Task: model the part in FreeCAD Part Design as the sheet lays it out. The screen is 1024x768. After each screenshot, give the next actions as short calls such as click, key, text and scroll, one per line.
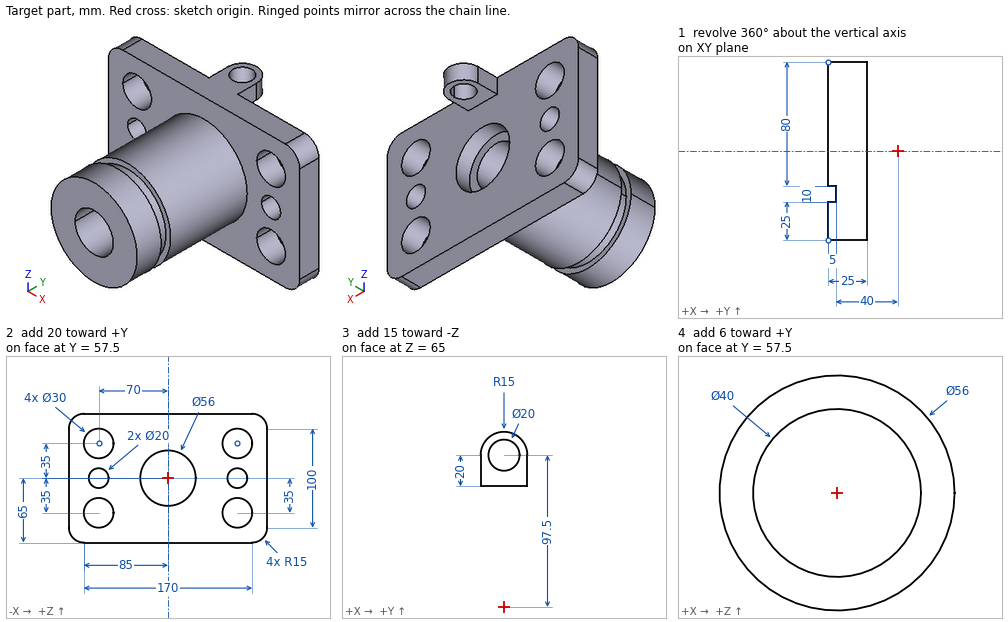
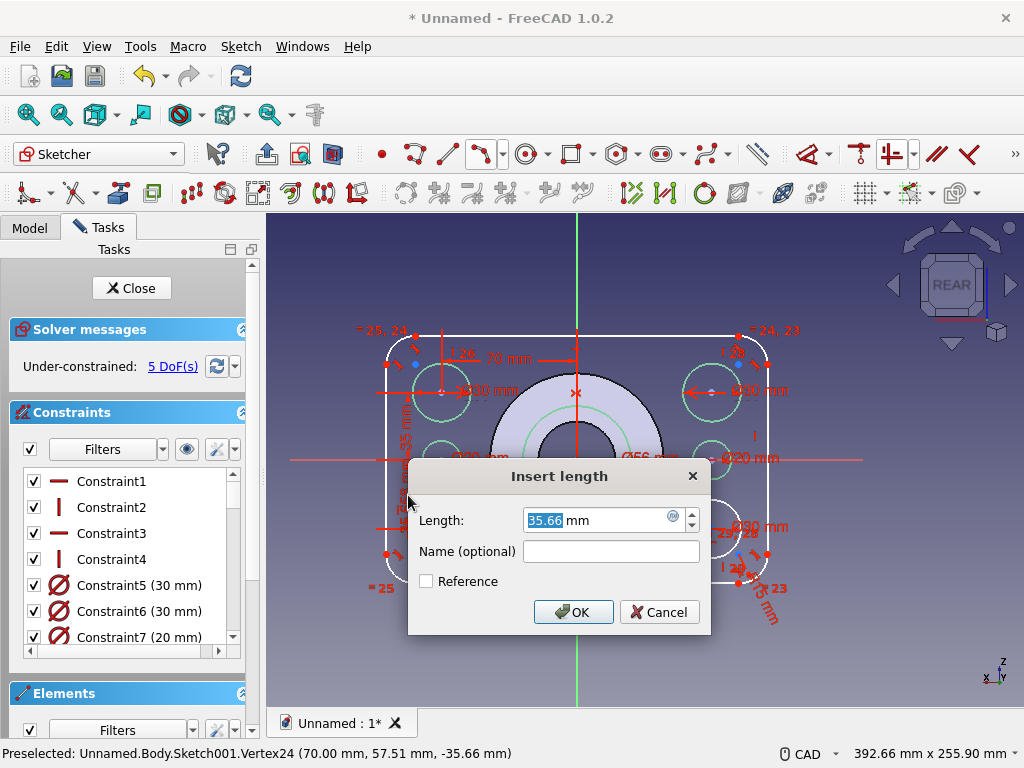
text(35)
key(Return)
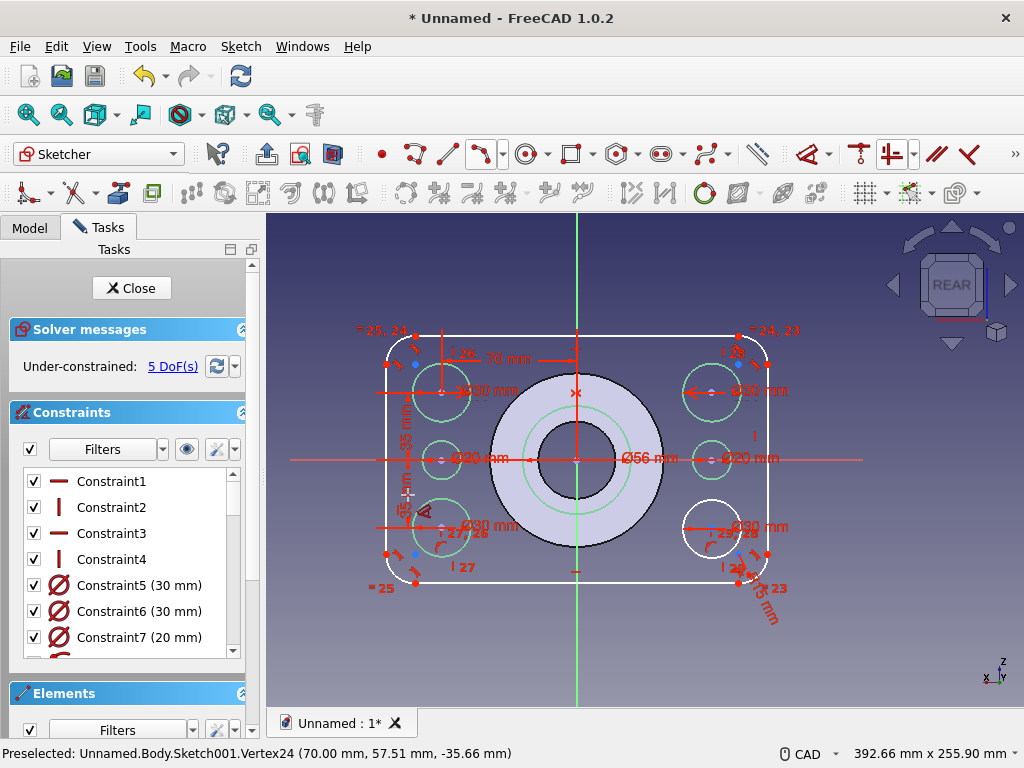
click(712, 529)
click(746, 495)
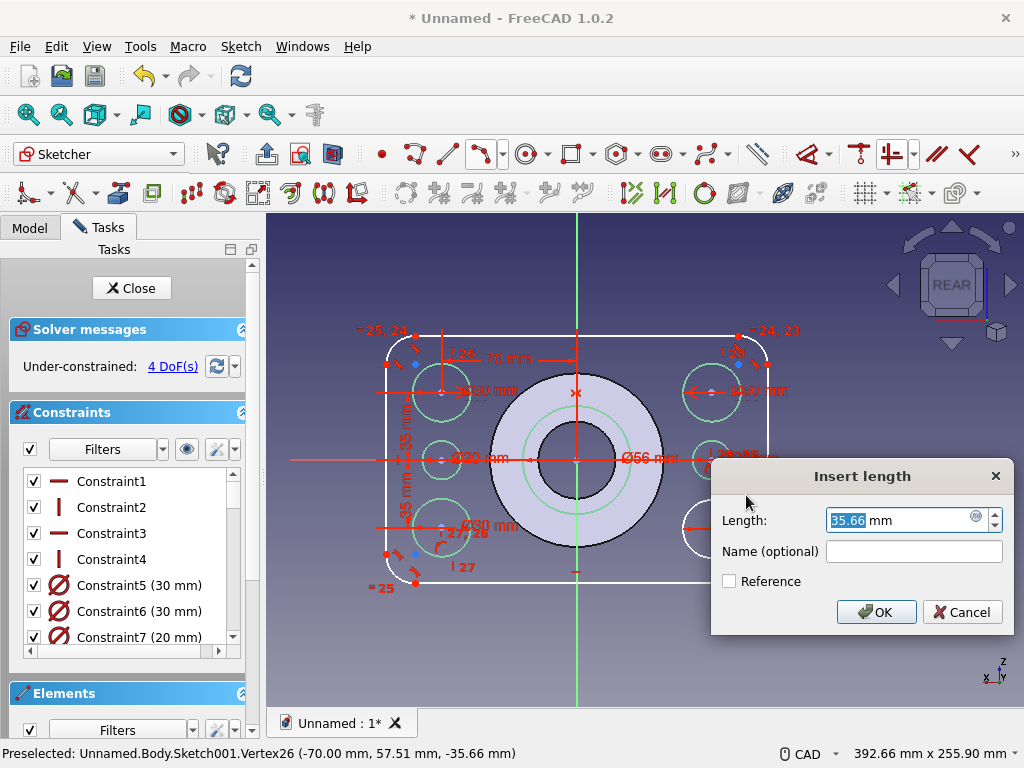
text(35)
key(Return)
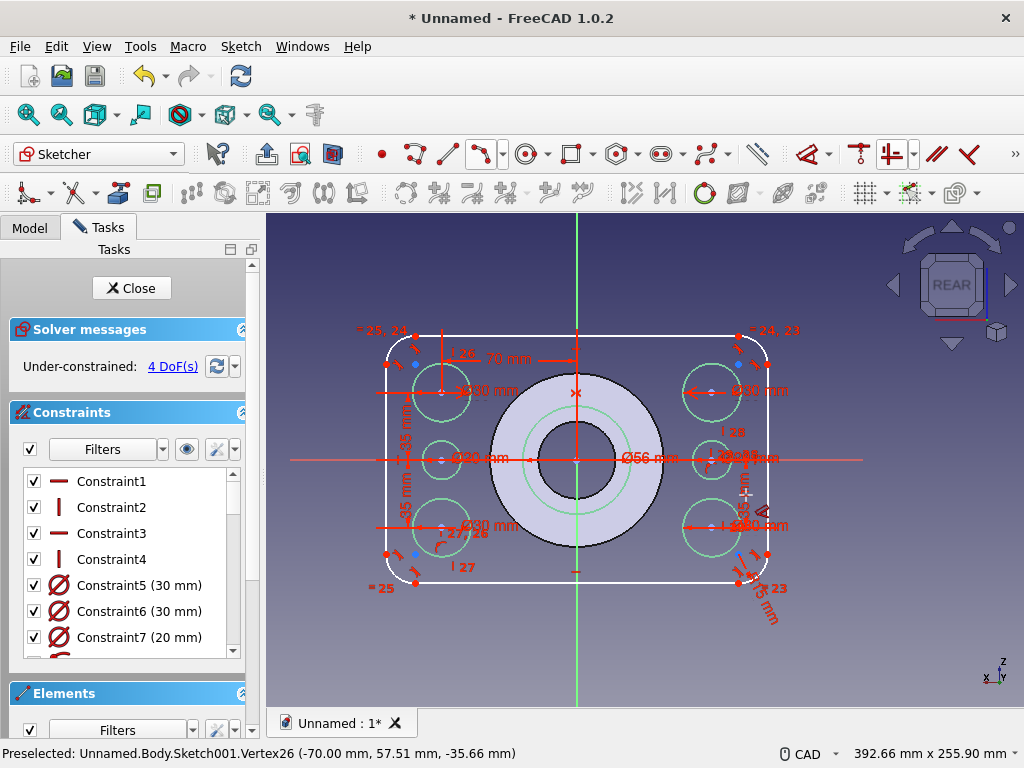
click(512, 583)
click(503, 617)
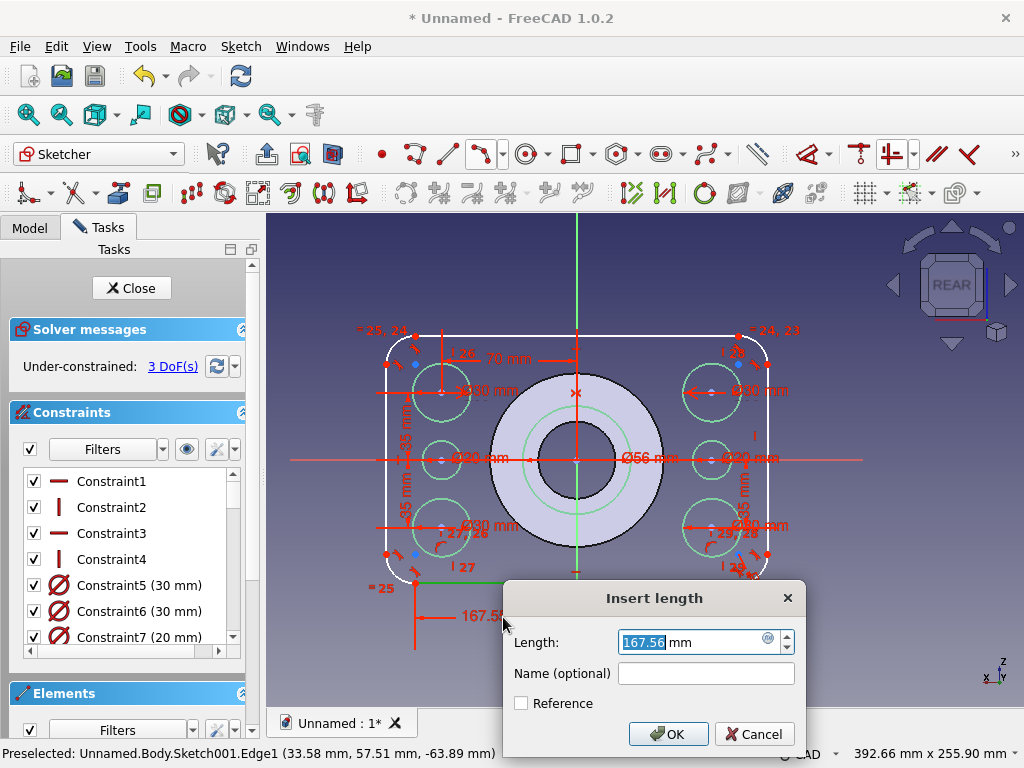
text(170)
key(Return)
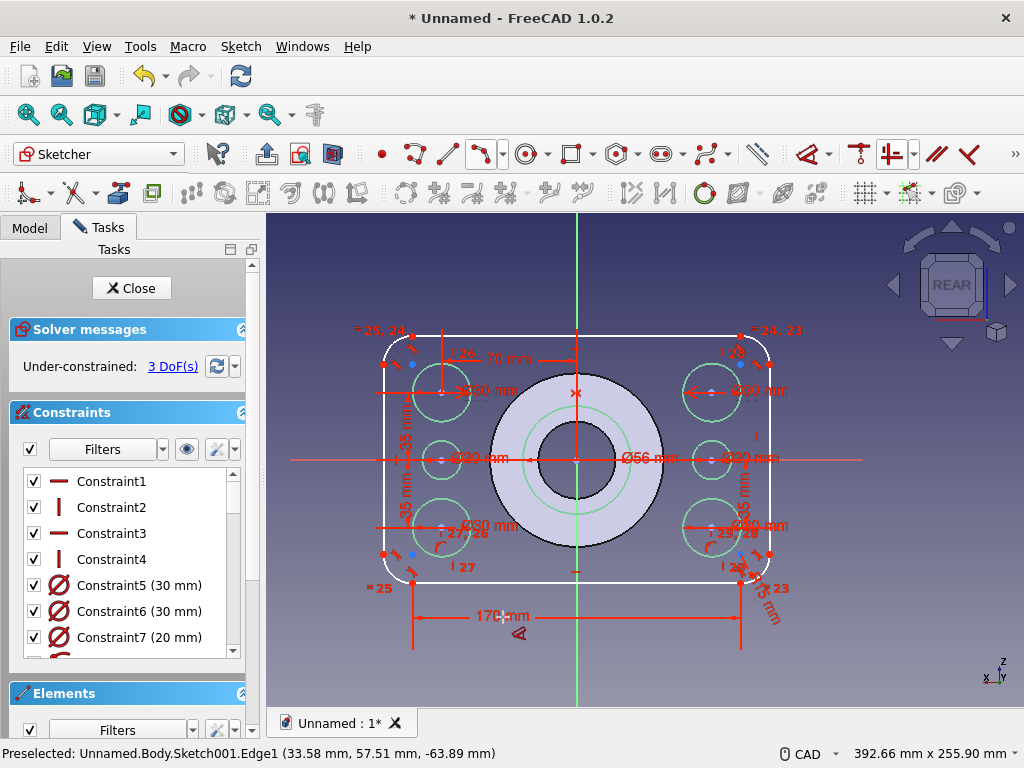
click(770, 498)
click(804, 416)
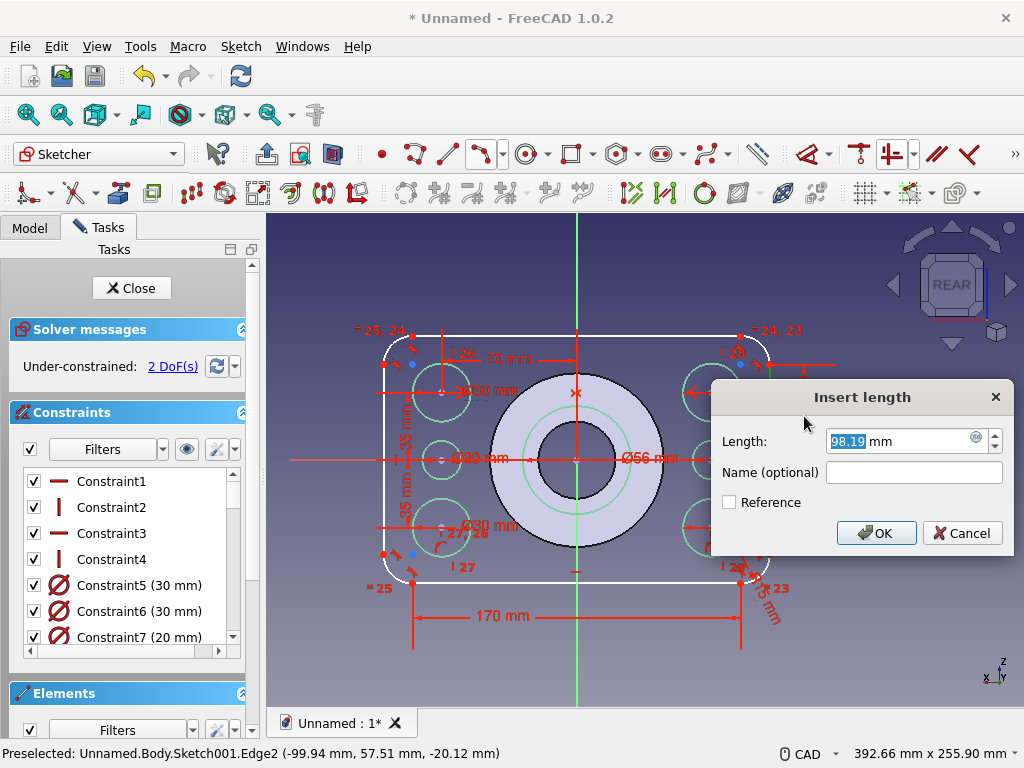
text(100)
key(Return)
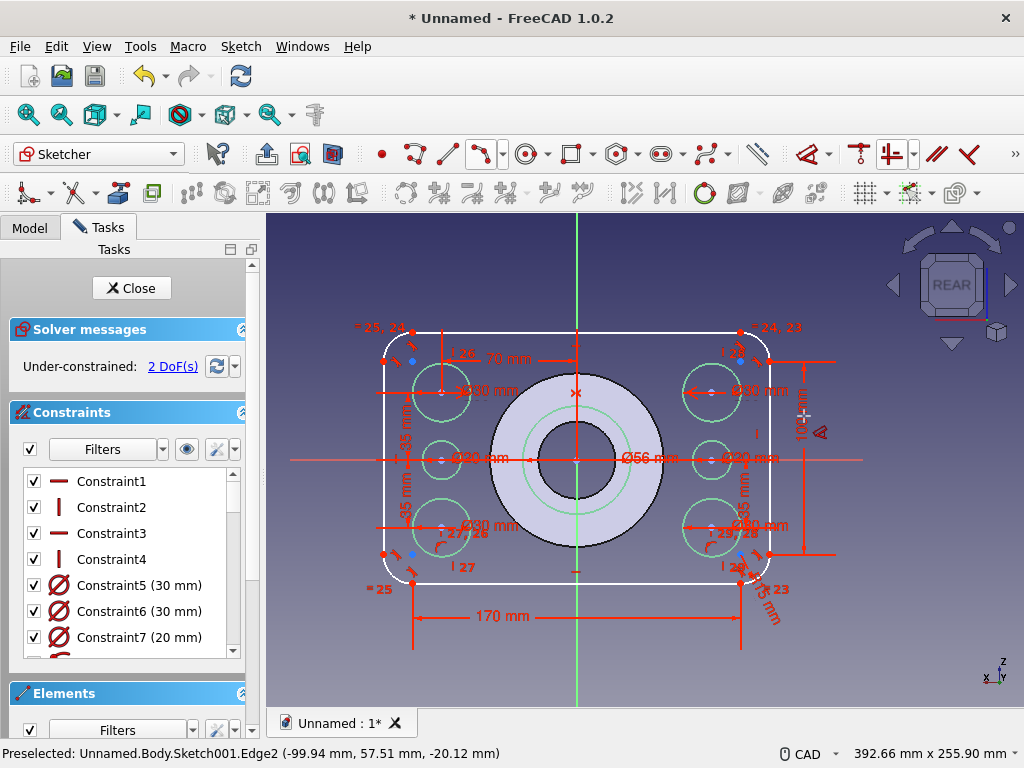
click(413, 584)
click(495, 426)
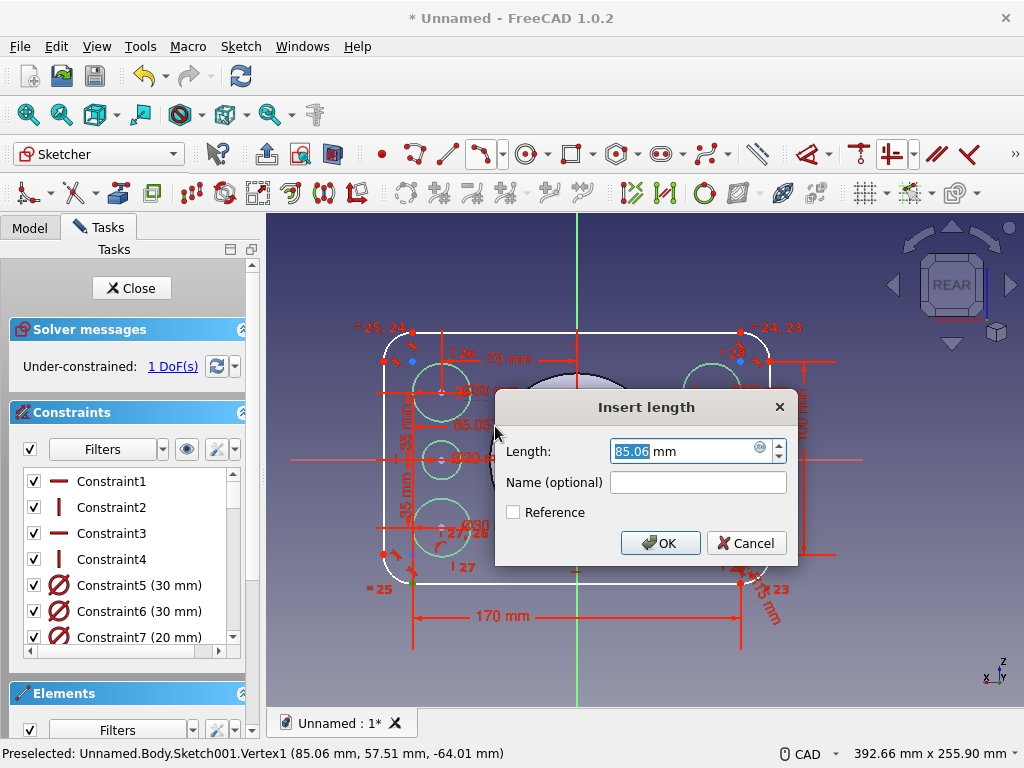
text(85)
key(Return)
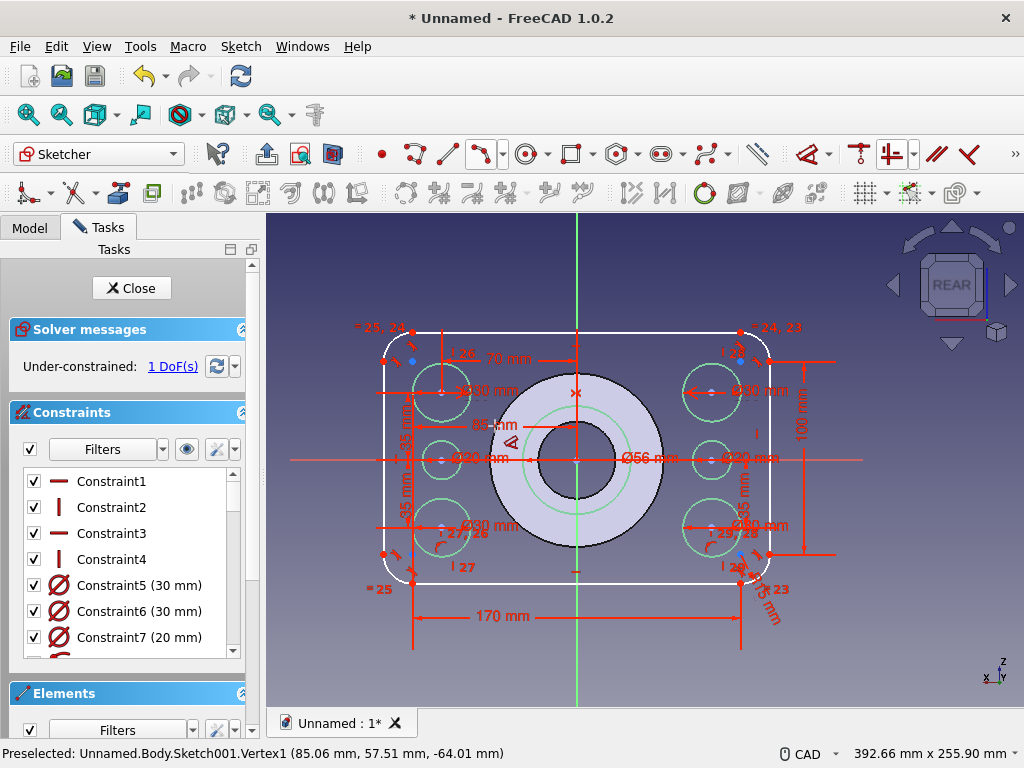
click(413, 584)
click(611, 522)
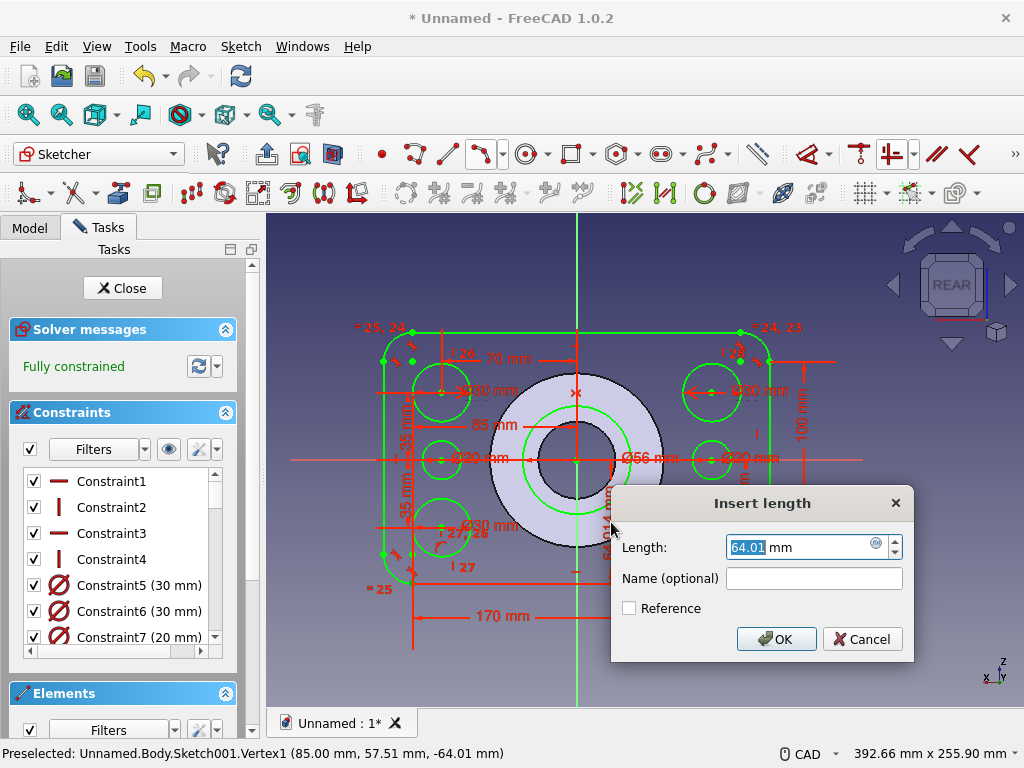
text(65)
key(Return)
key(Escape)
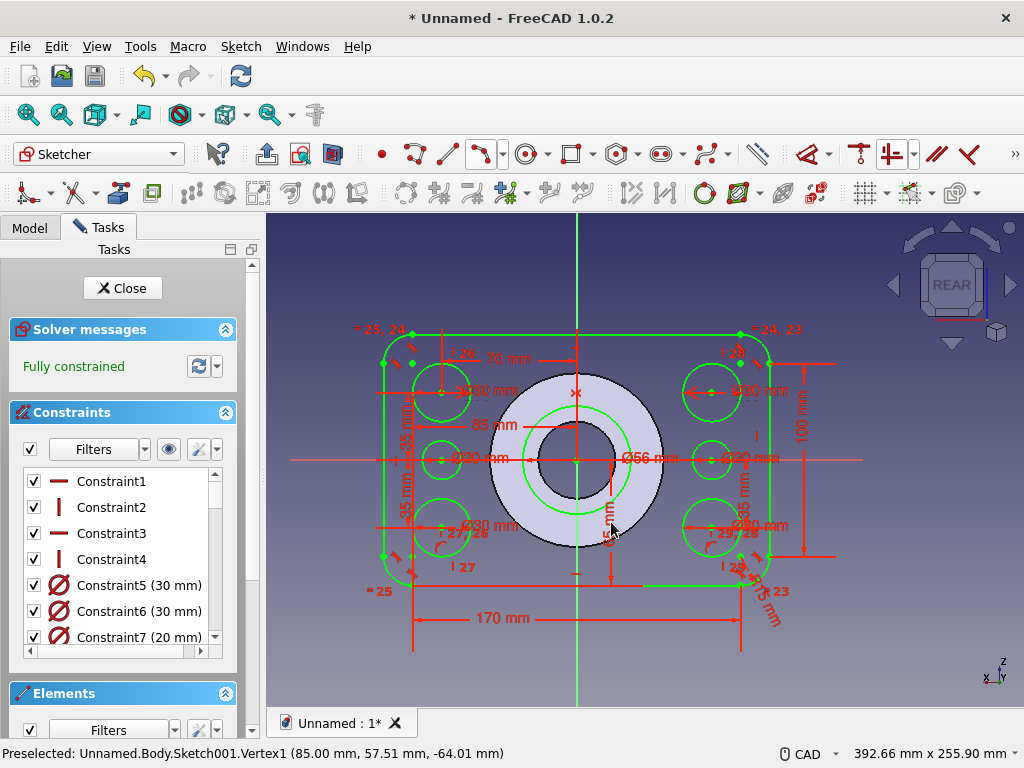
click(123, 288)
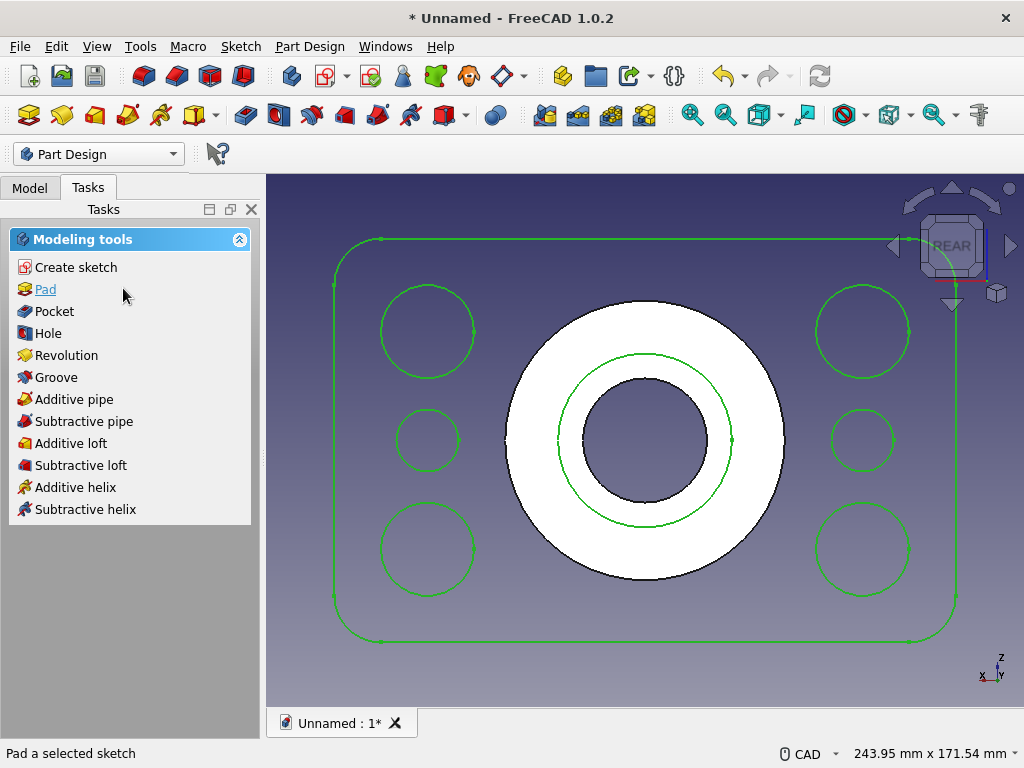
click(29, 116)